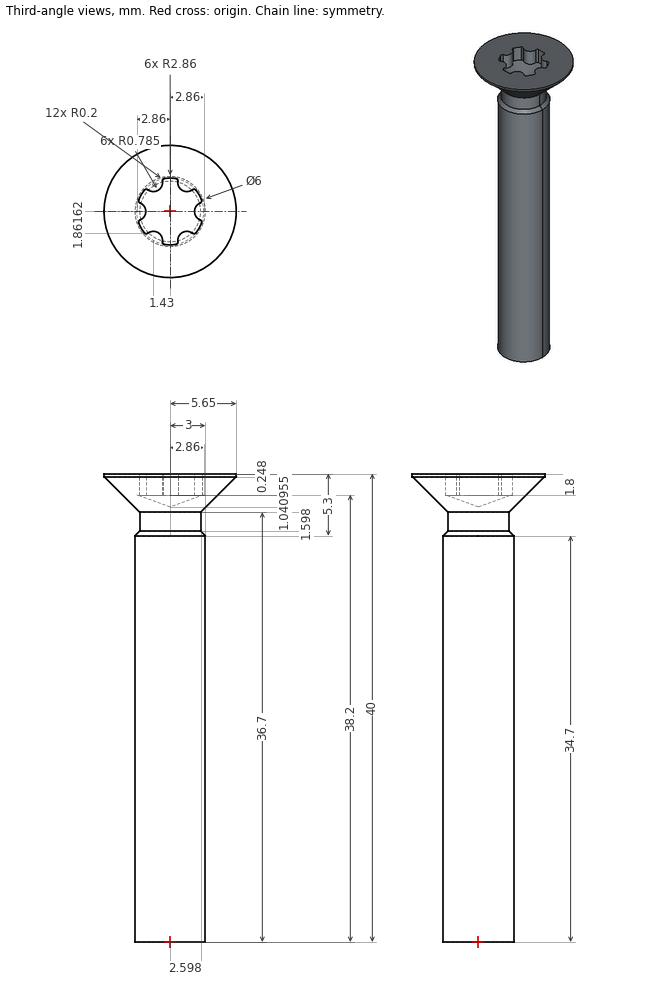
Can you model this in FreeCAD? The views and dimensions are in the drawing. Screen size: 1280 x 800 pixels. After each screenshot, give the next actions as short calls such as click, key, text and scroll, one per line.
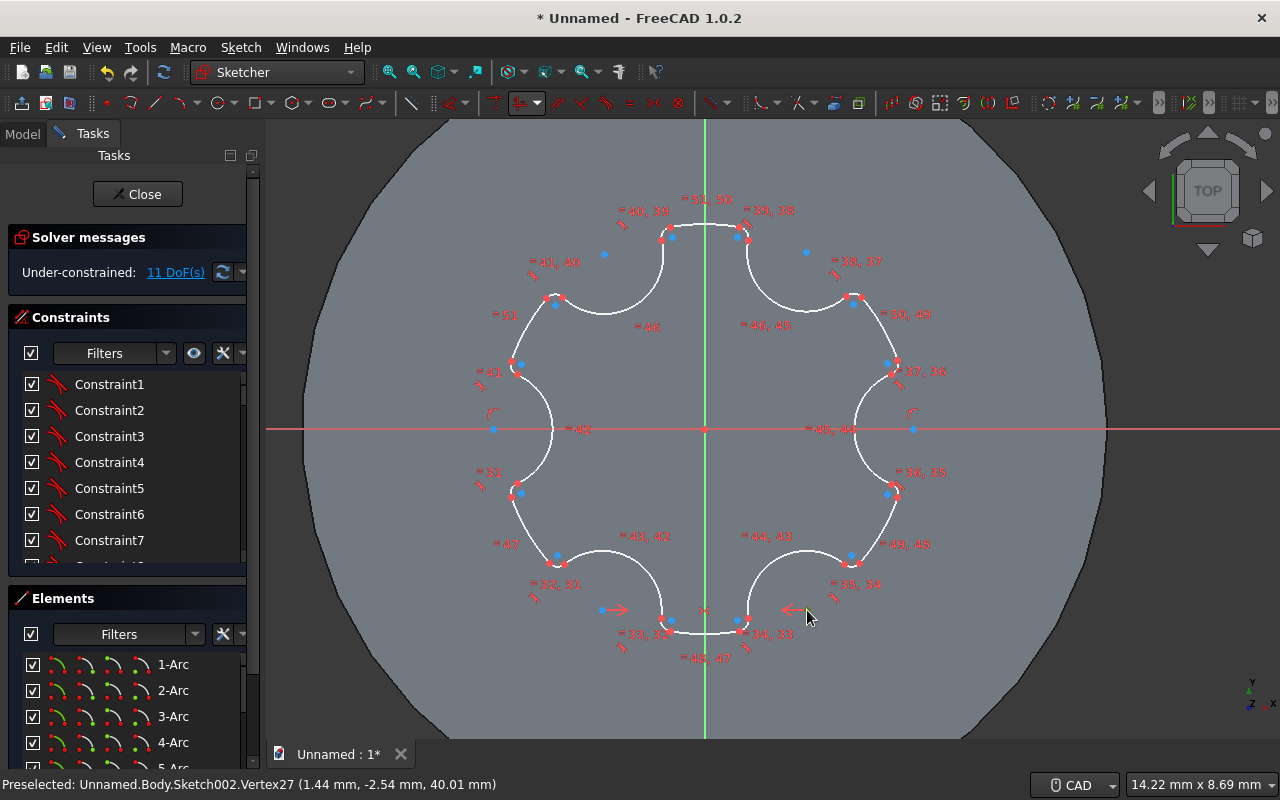
click(806, 252)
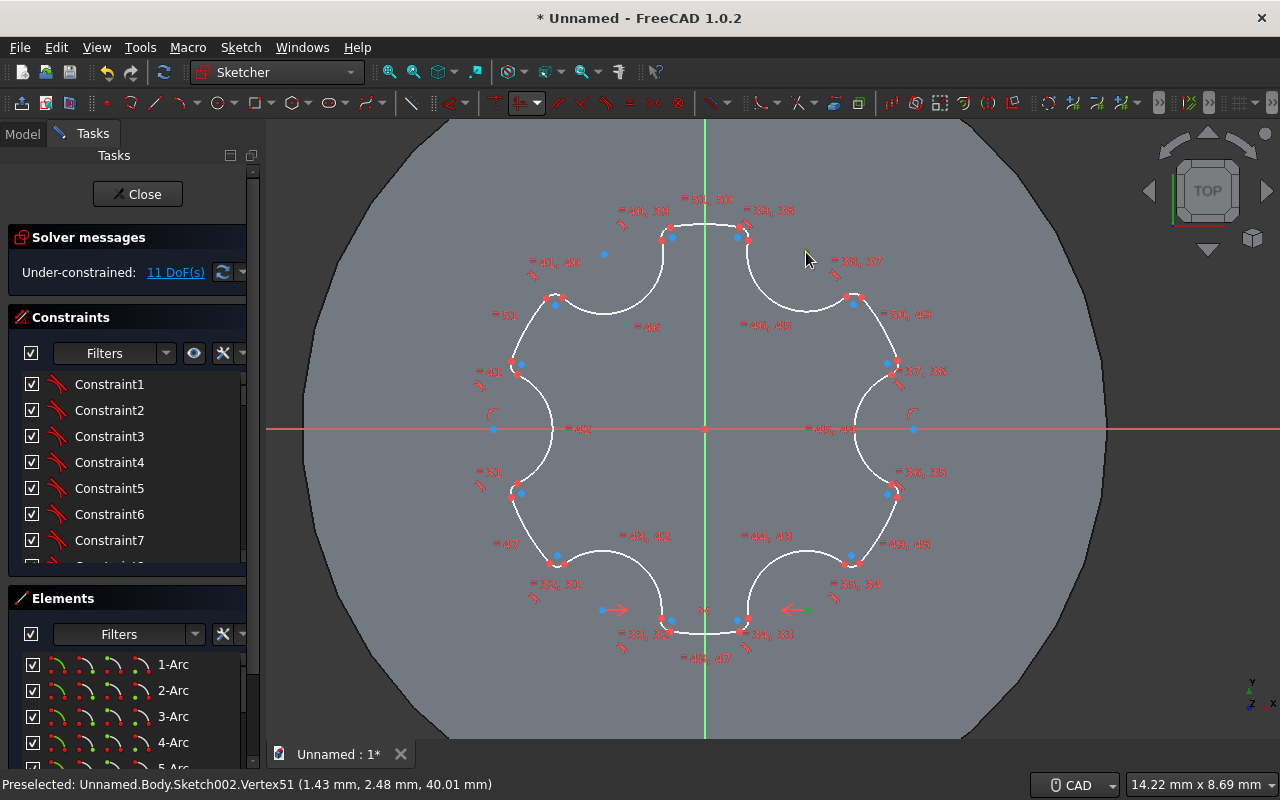
click(353, 429)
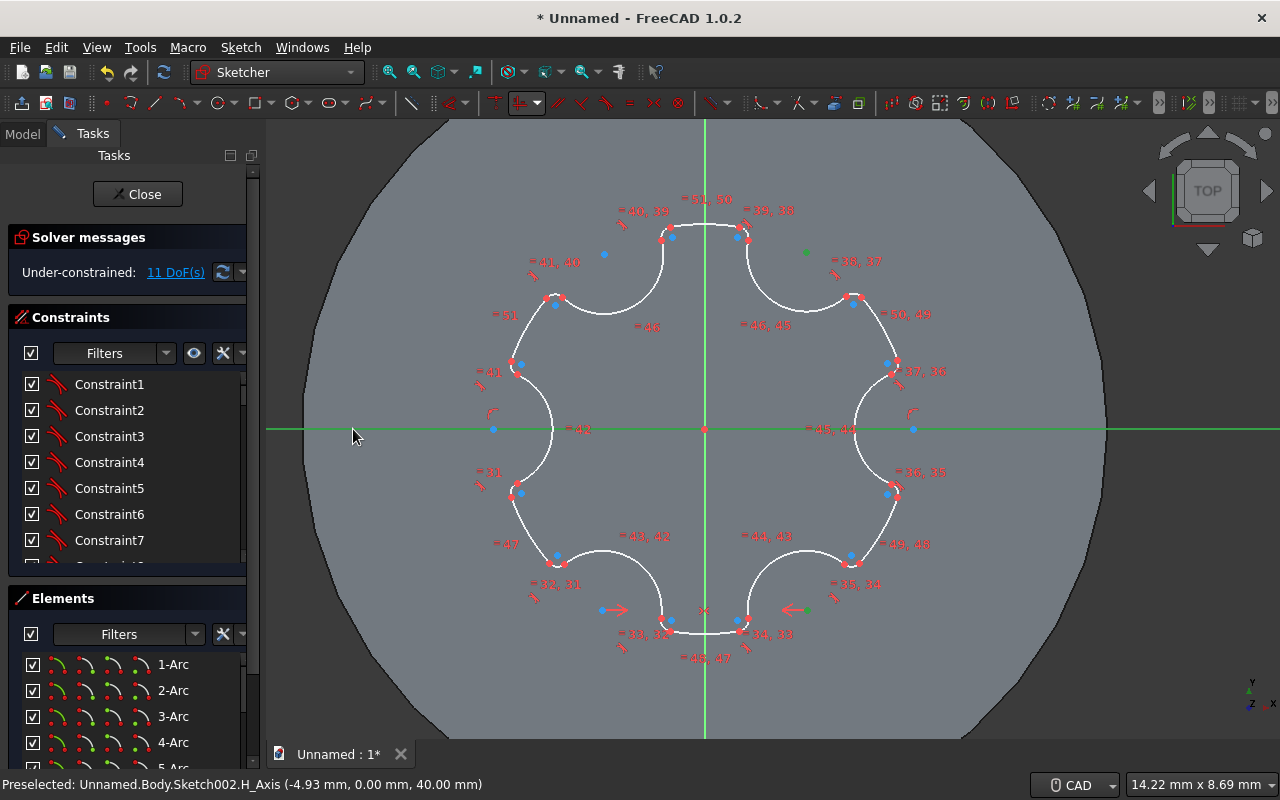
click(654, 104)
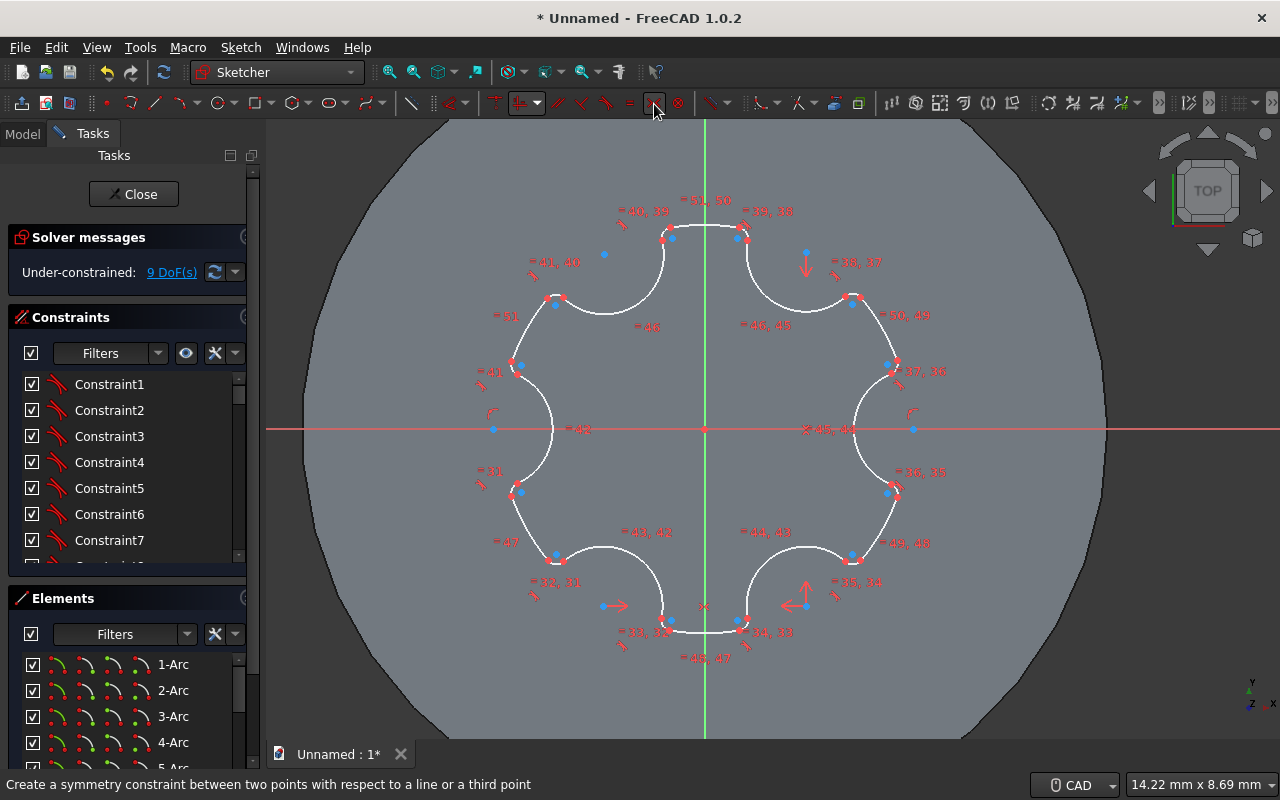
click(603, 606)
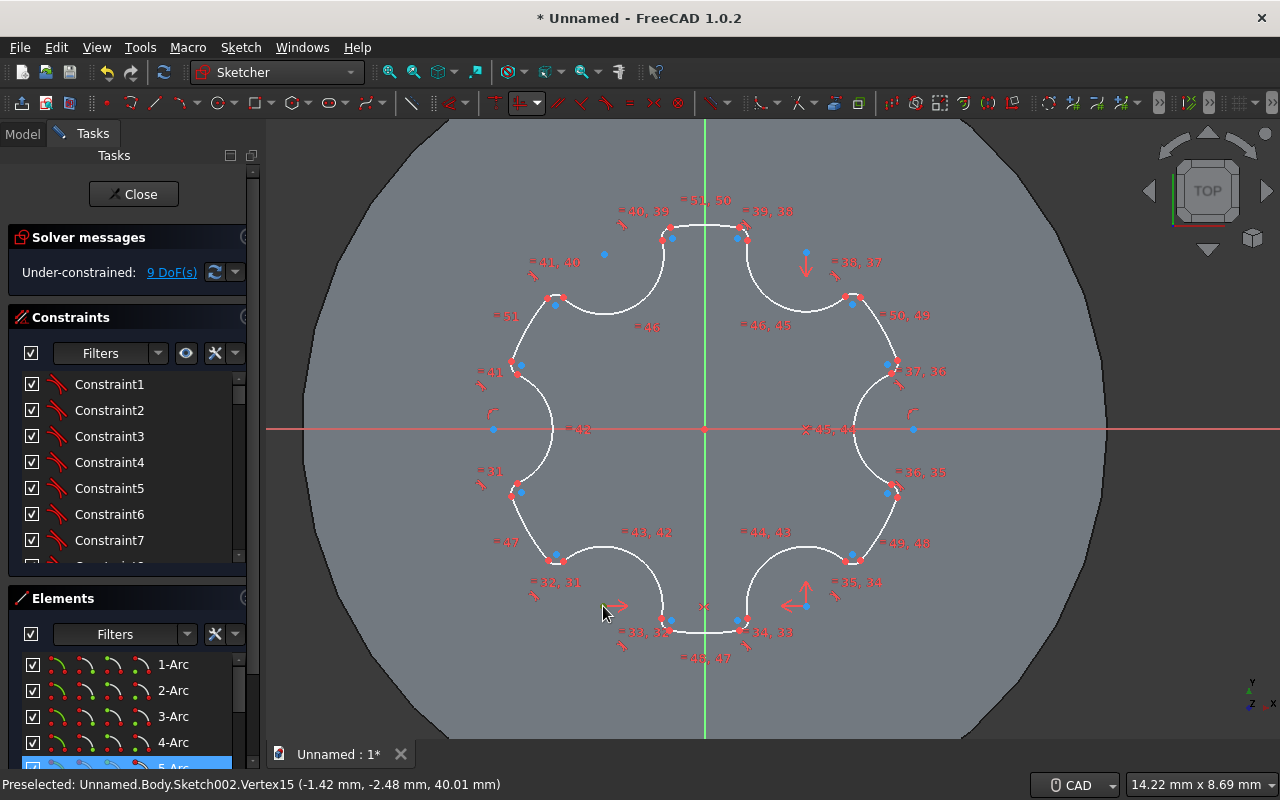
click(604, 255)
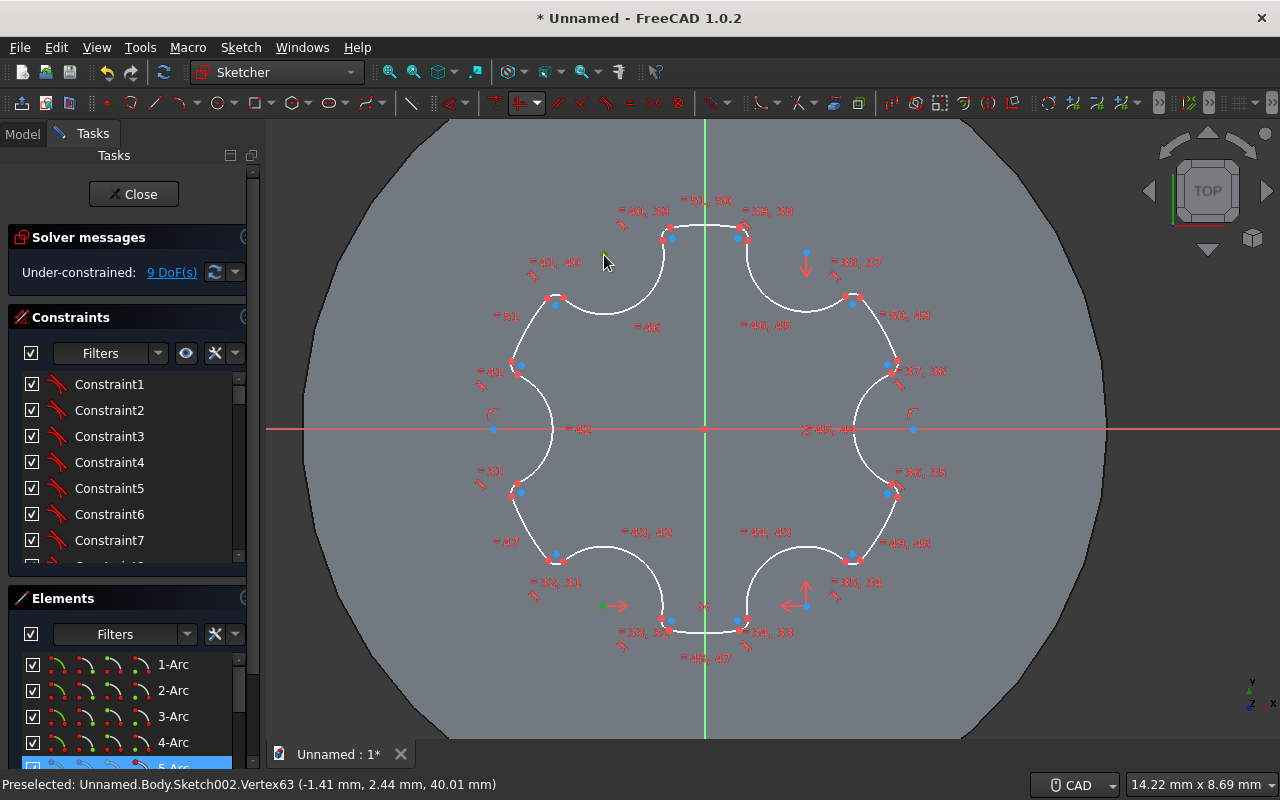
click(353, 429)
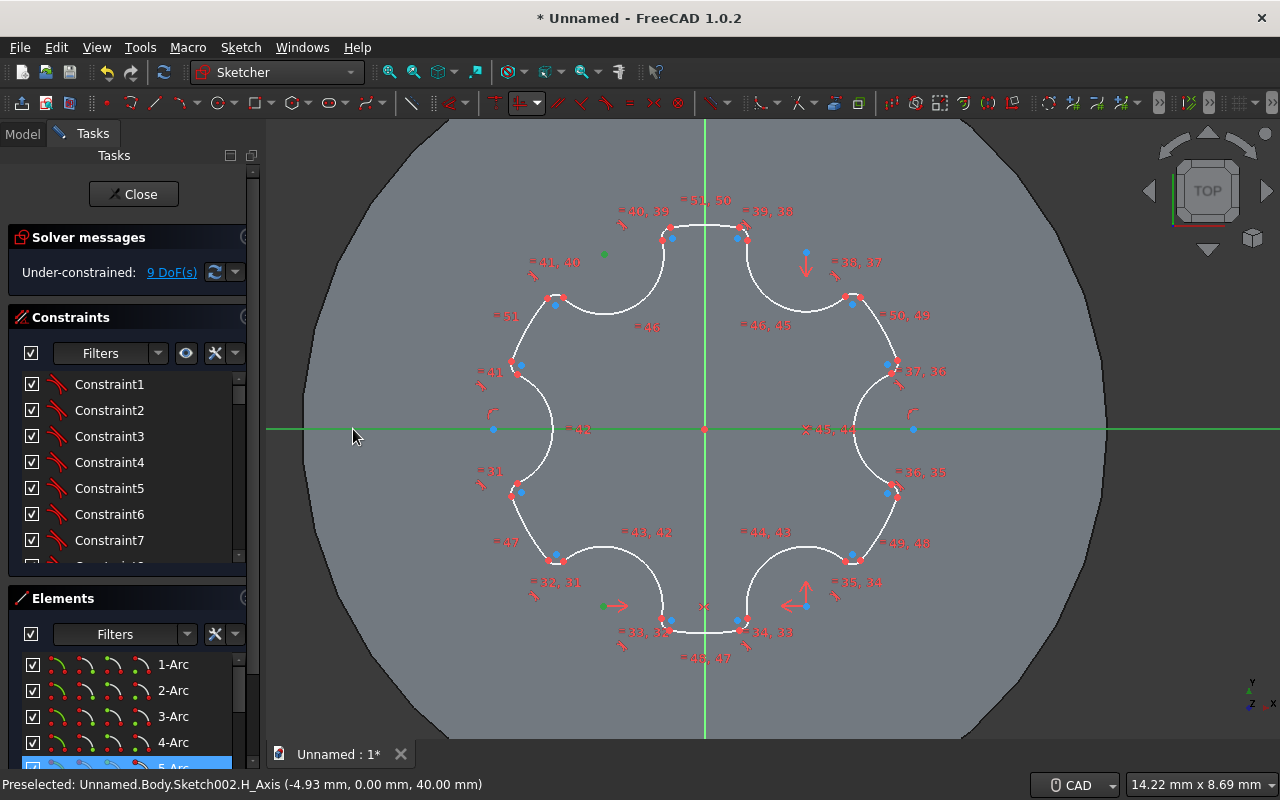
key(s)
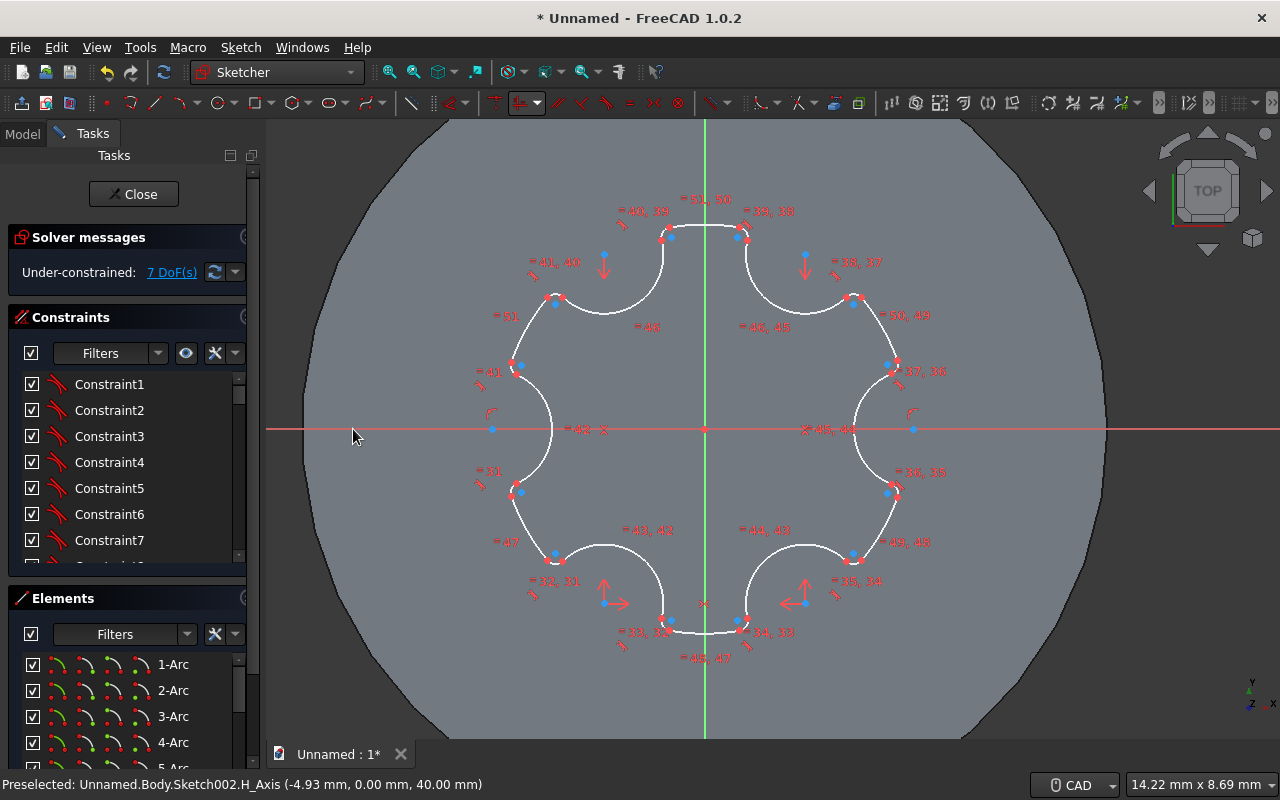
click(546, 455)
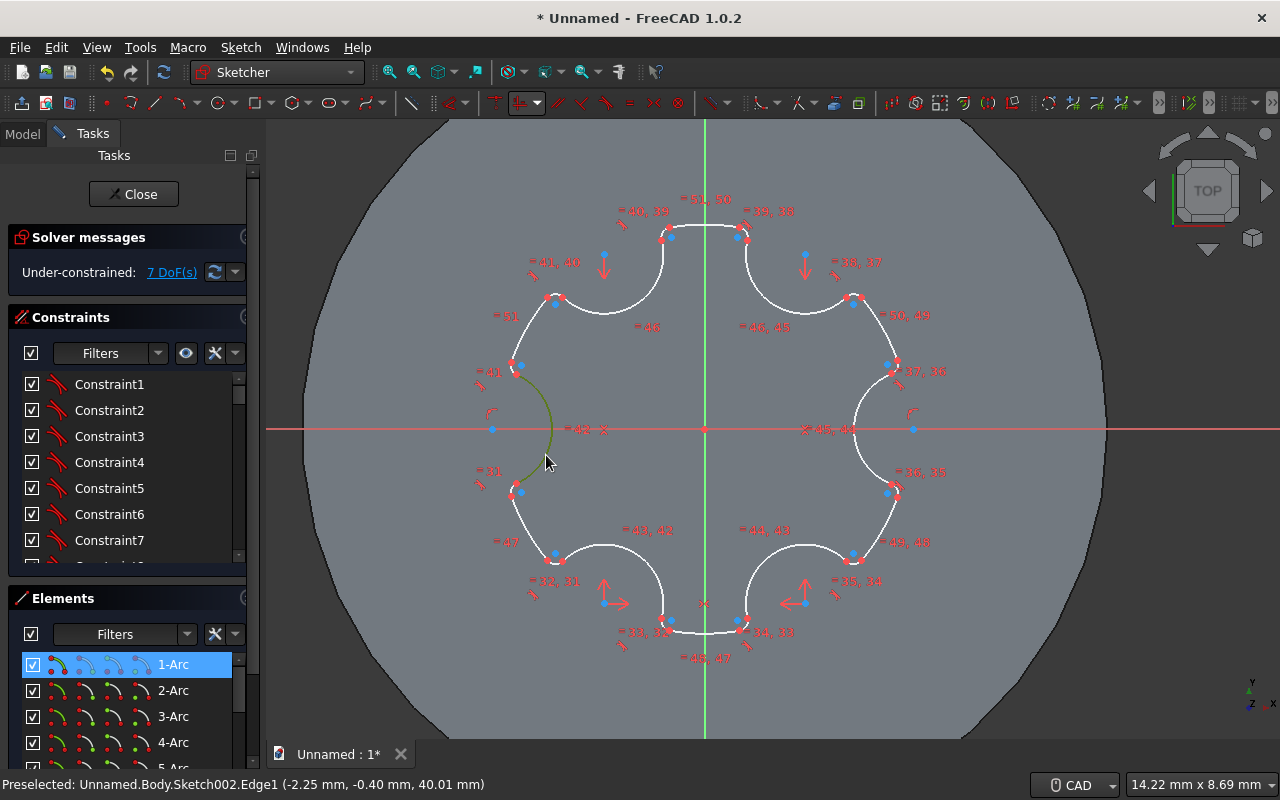
key(k)
key(r)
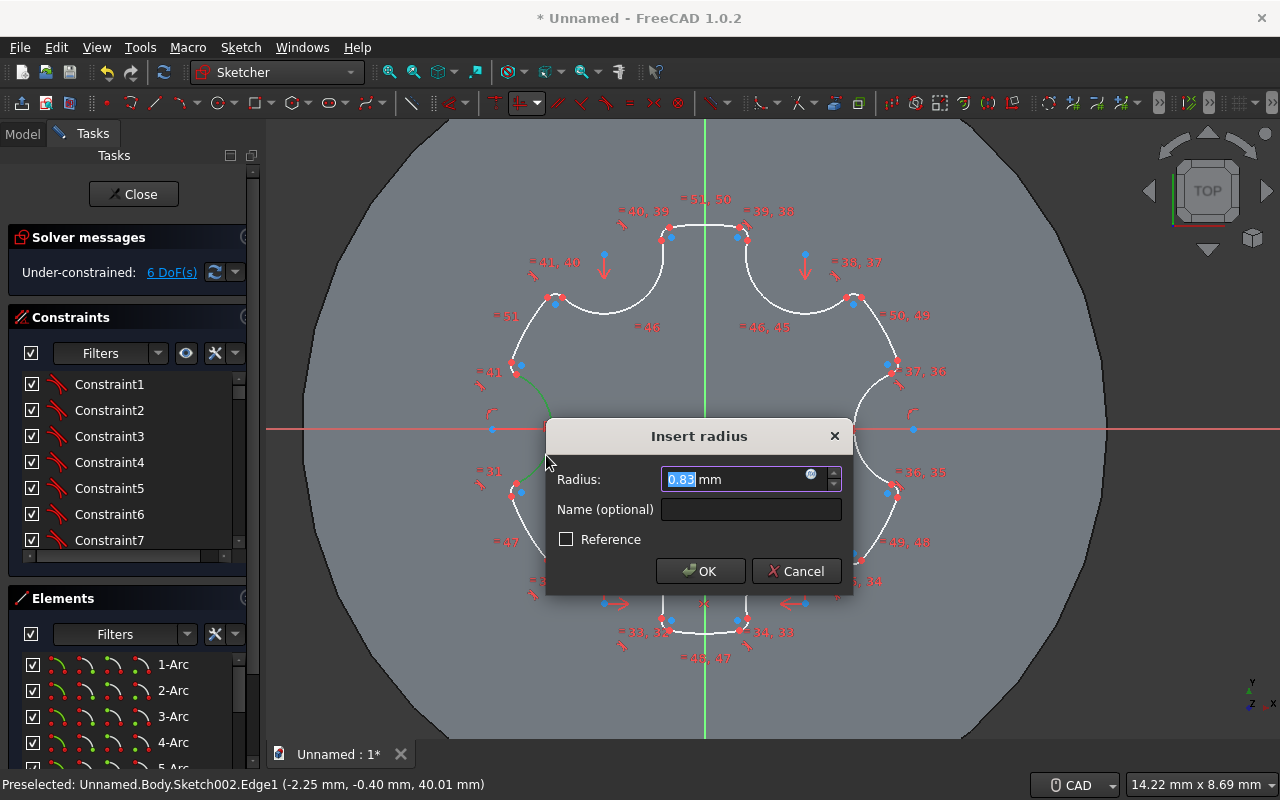
text(0.785)
key(Return)